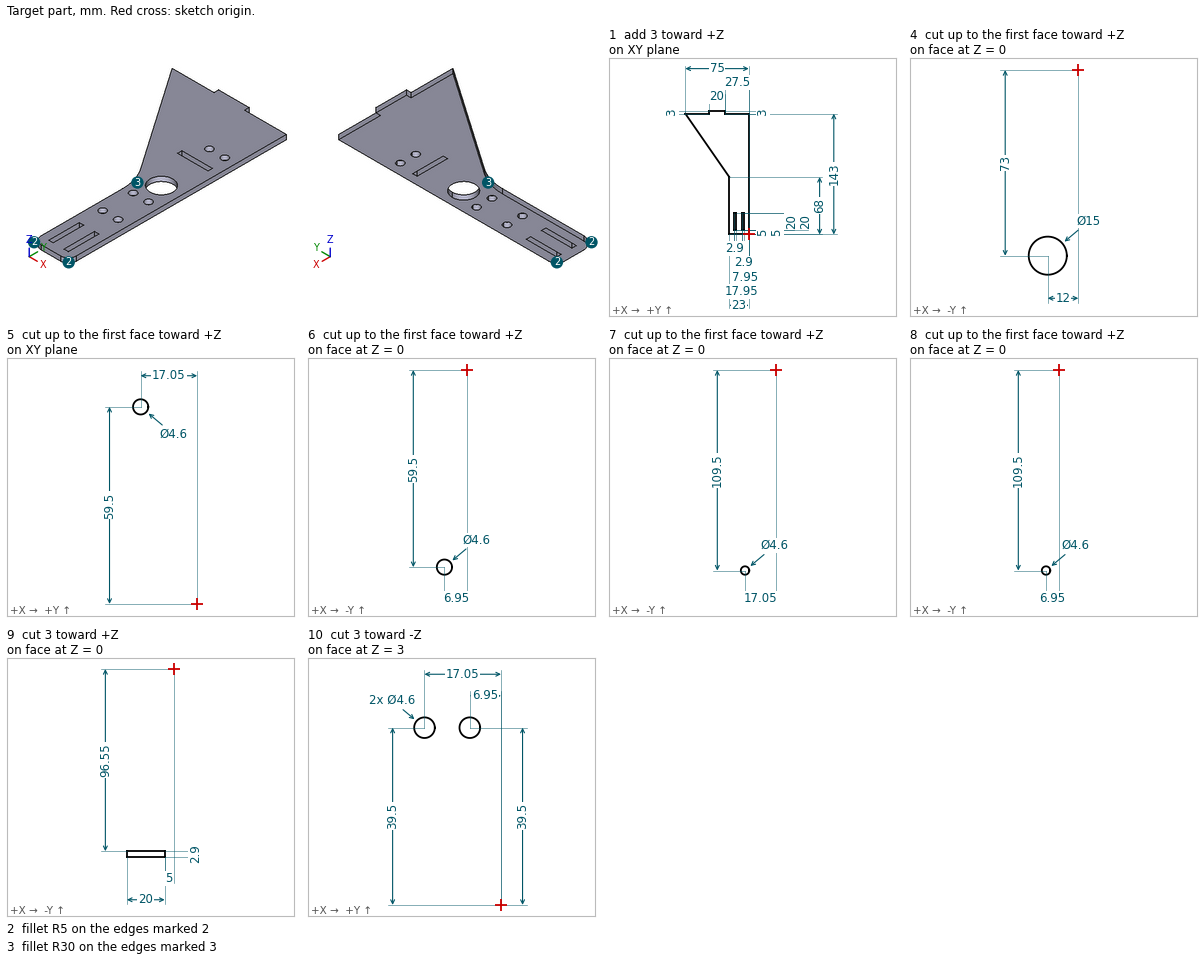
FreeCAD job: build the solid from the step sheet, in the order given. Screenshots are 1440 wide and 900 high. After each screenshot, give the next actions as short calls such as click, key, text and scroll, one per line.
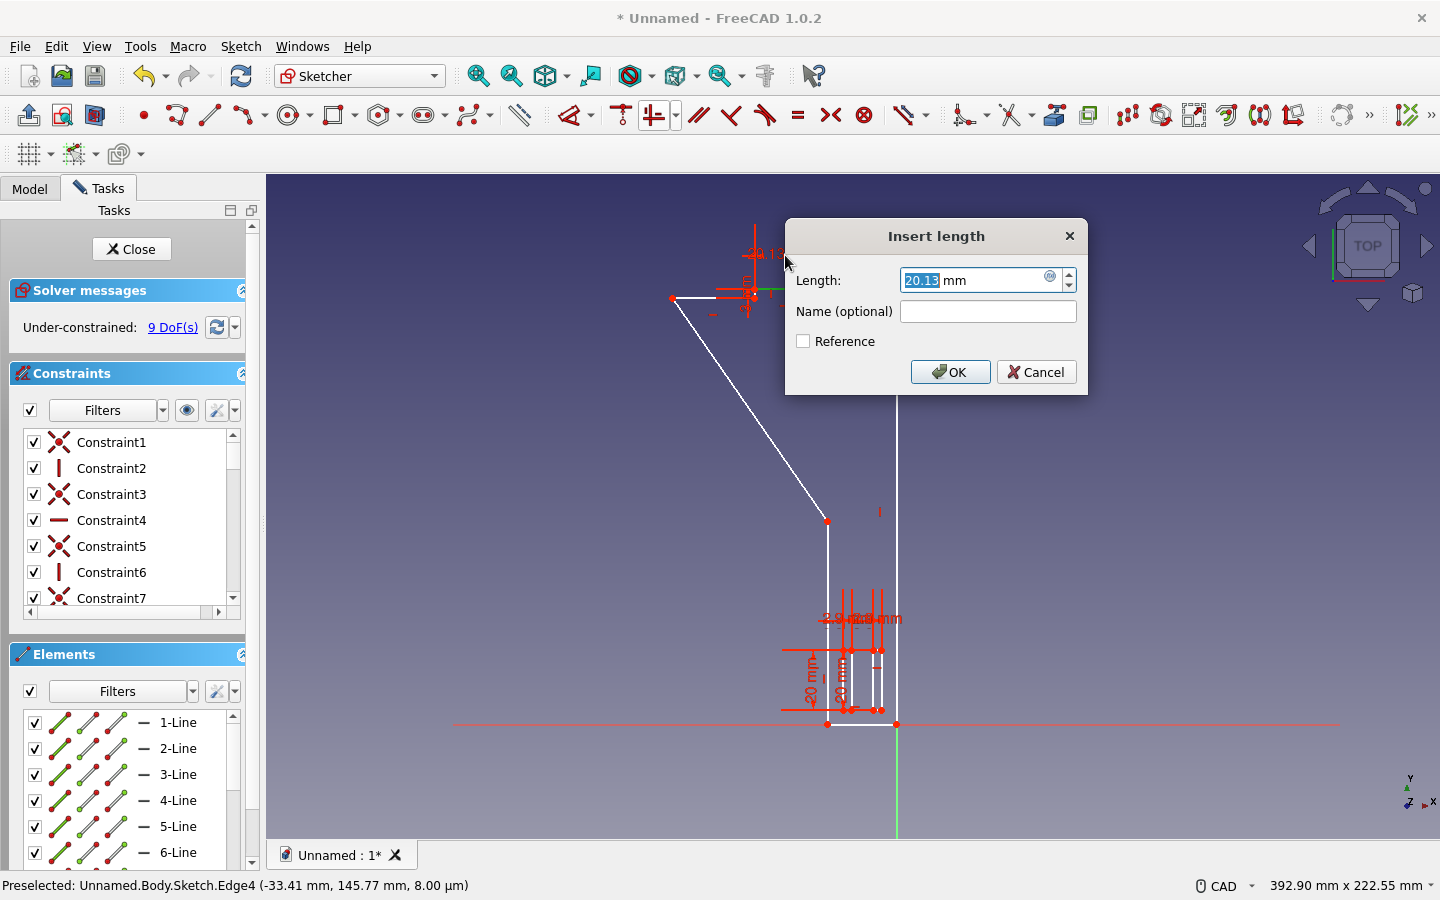
text(20)
key(Return)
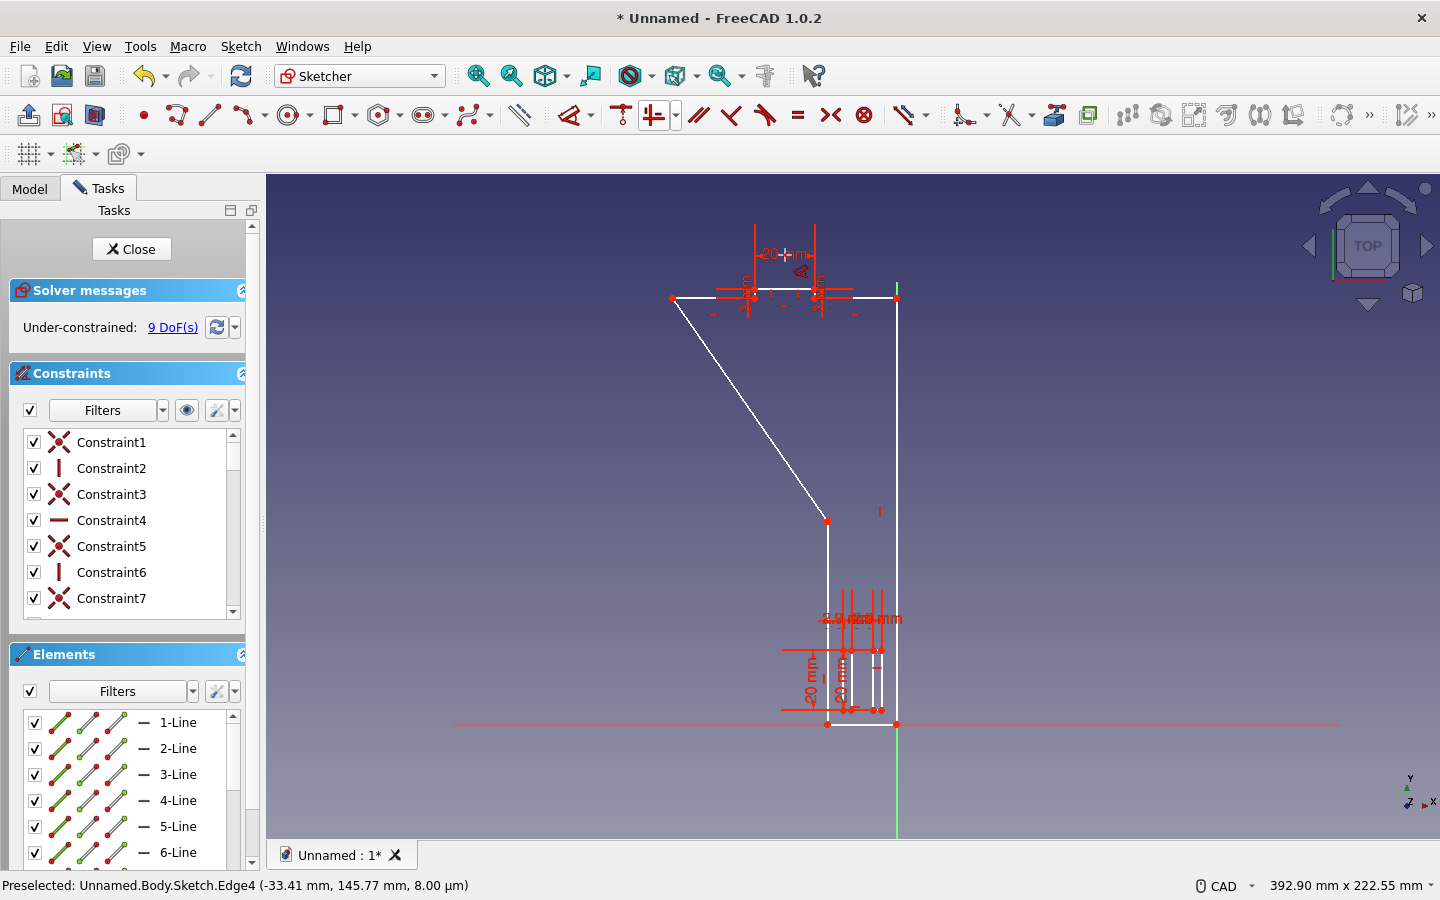
click(828, 583)
click(862, 623)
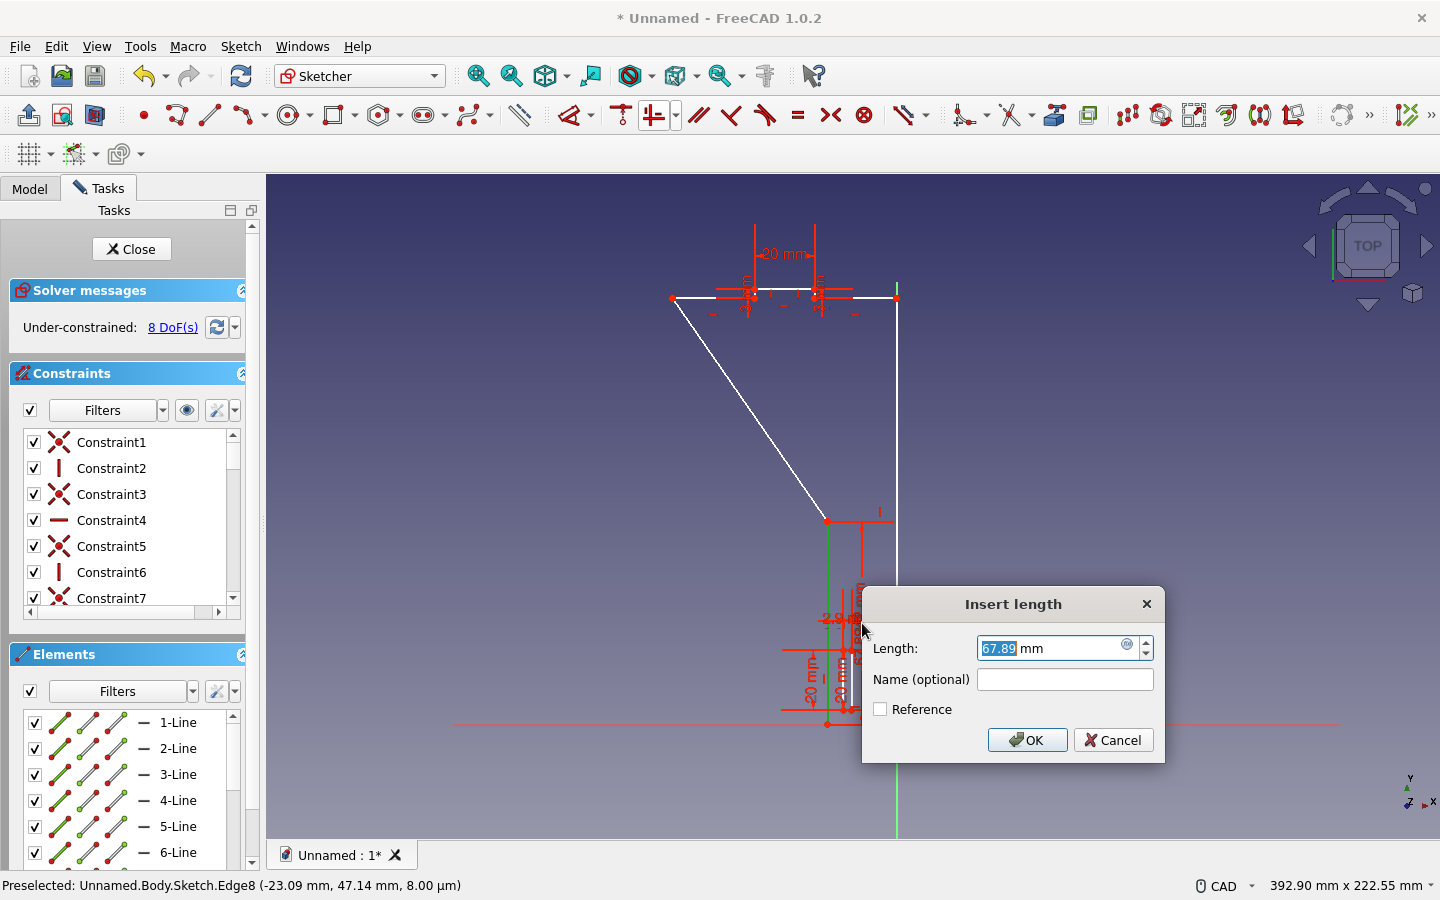
text(68)
key(Return)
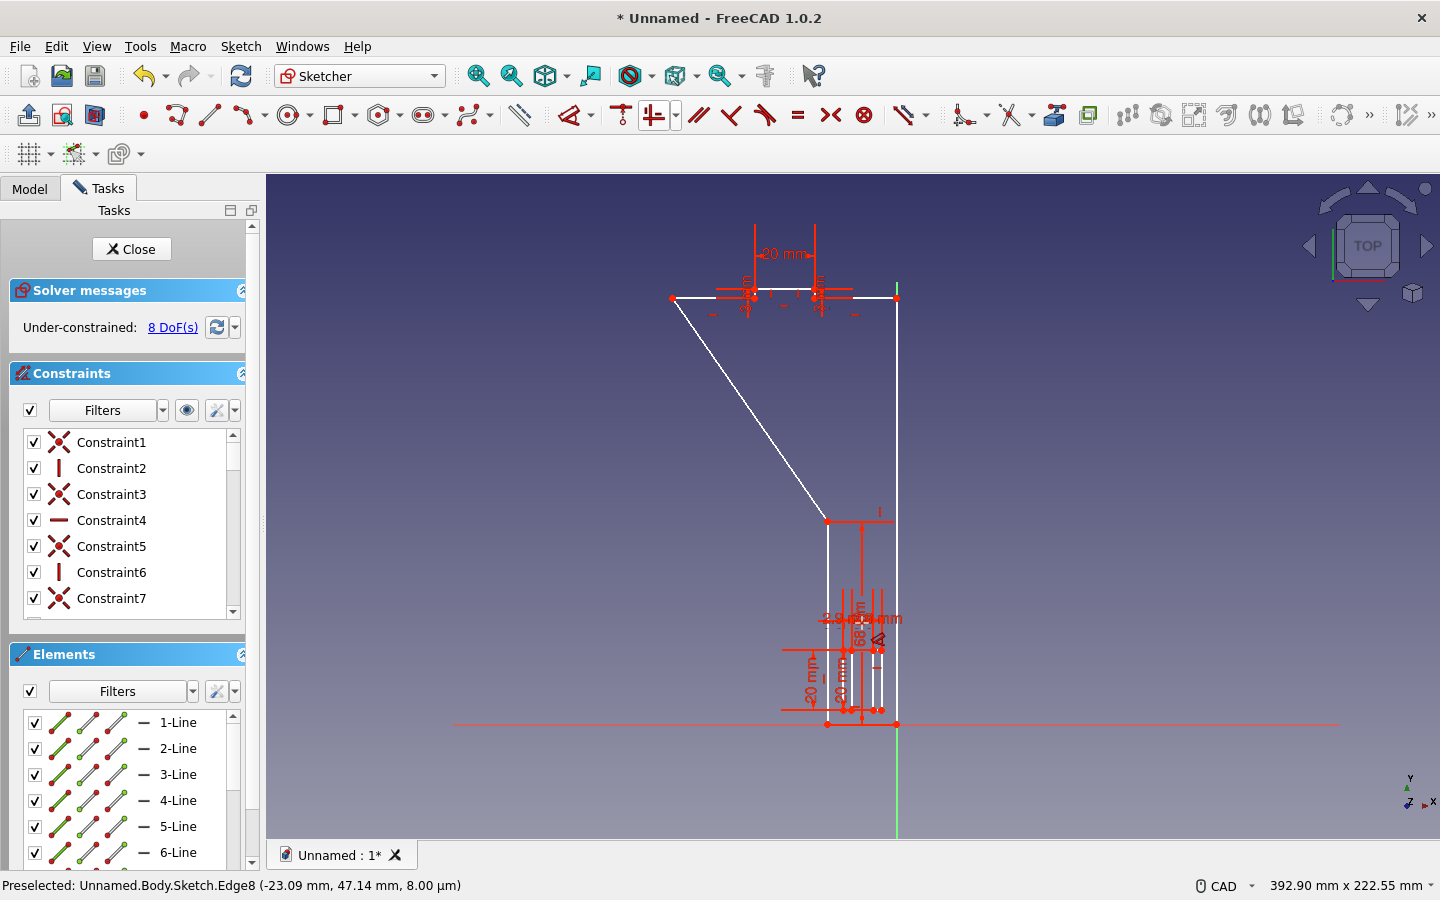
click(849, 725)
click(862, 759)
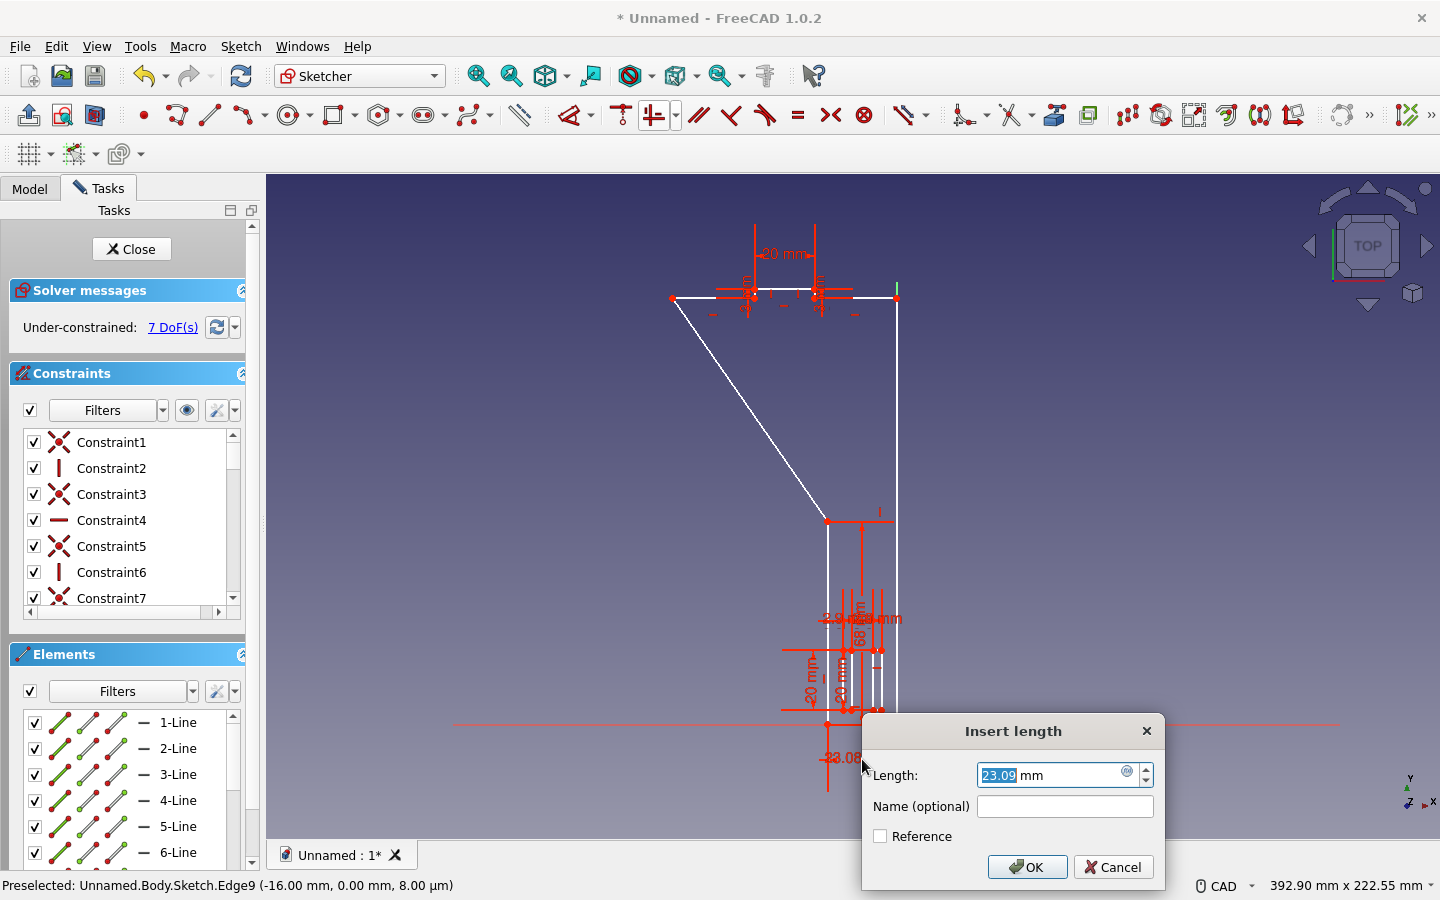
text(23)
key(Return)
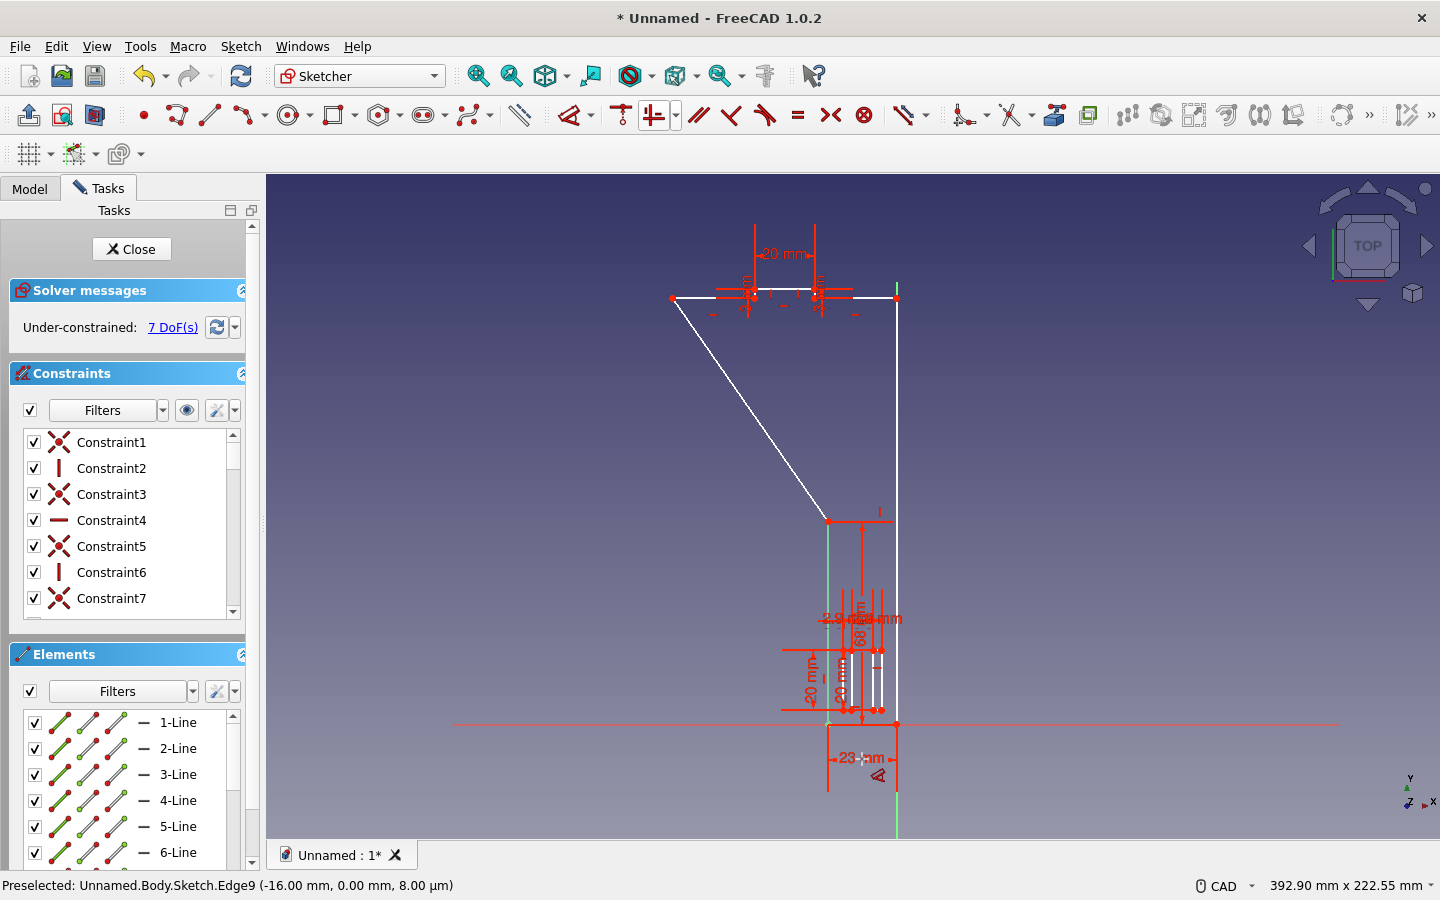
scroll(873, 710, up, 5)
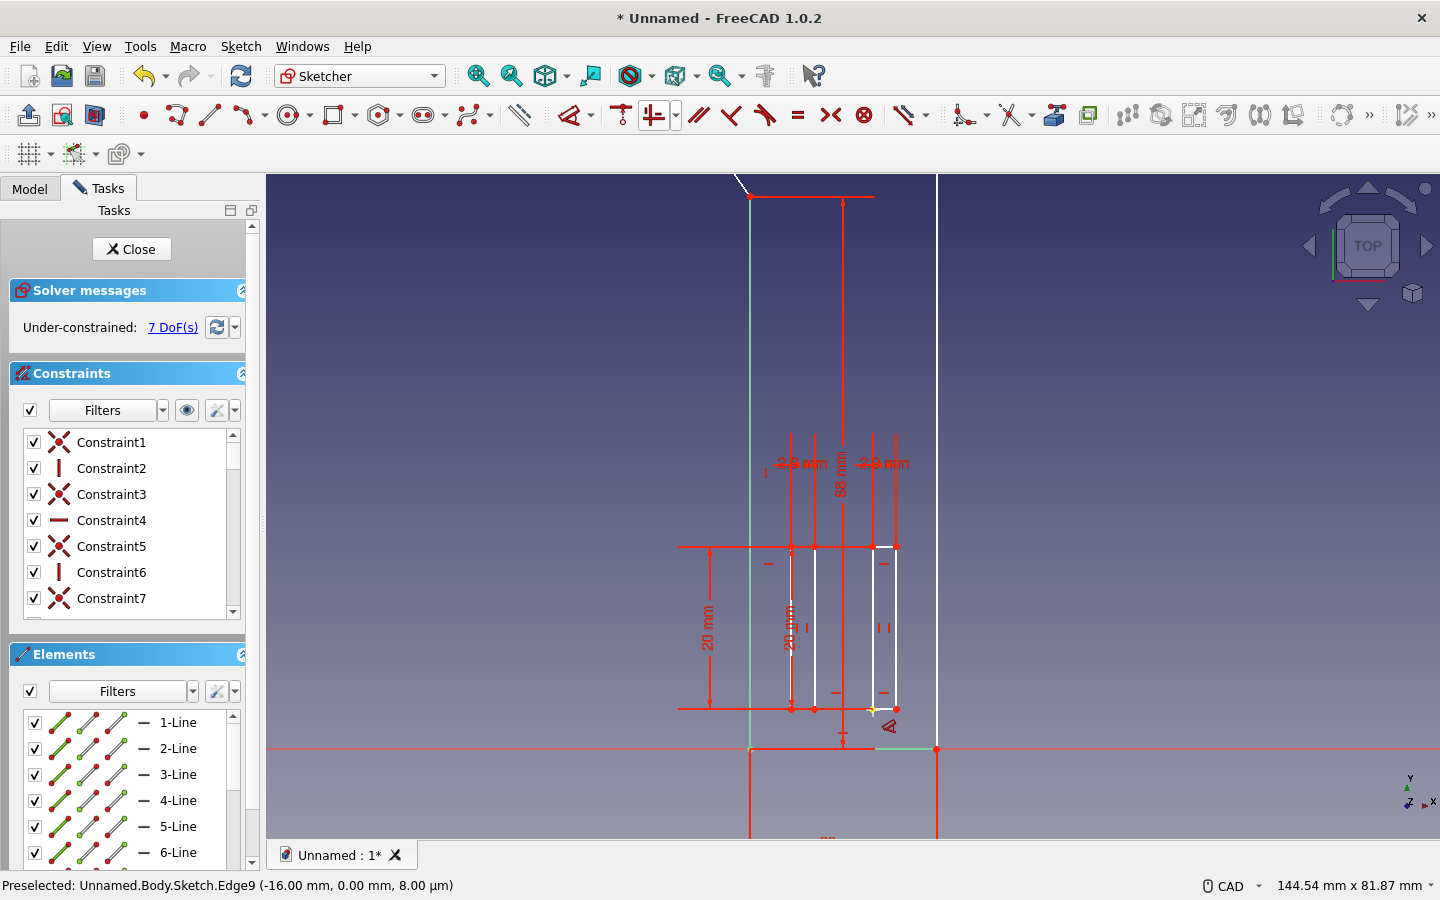
click(873, 709)
click(971, 729)